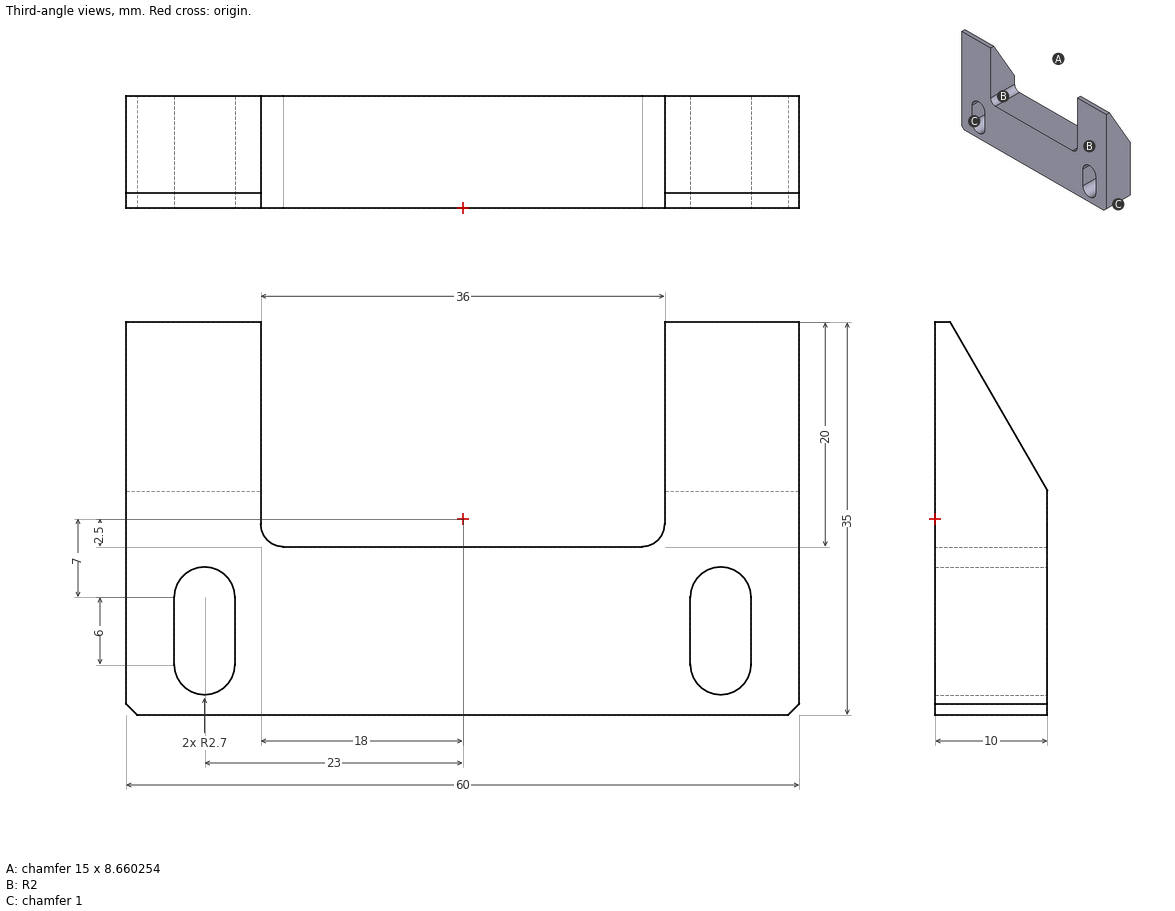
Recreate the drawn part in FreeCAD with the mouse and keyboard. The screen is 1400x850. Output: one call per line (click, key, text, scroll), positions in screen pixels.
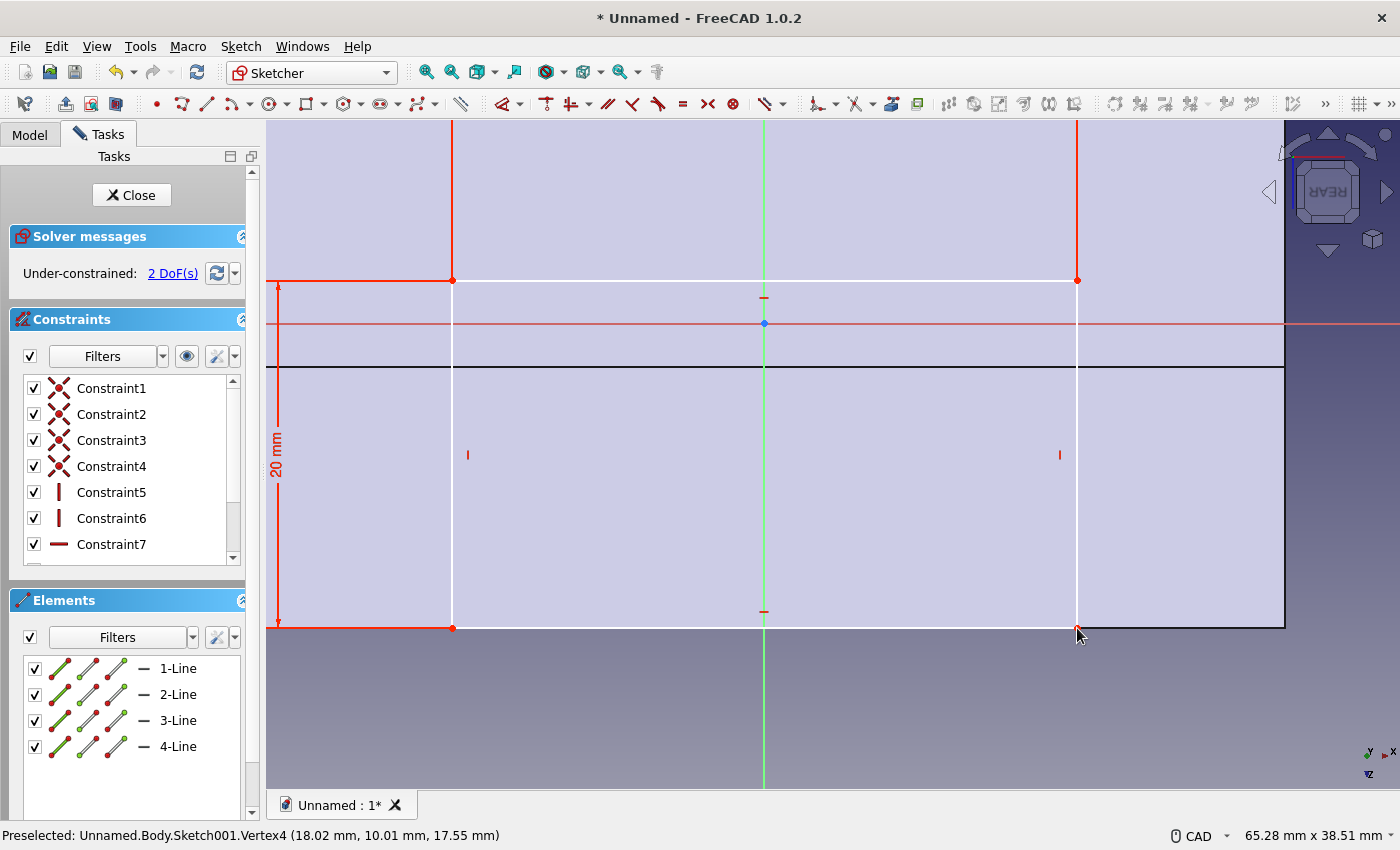
click(502, 104)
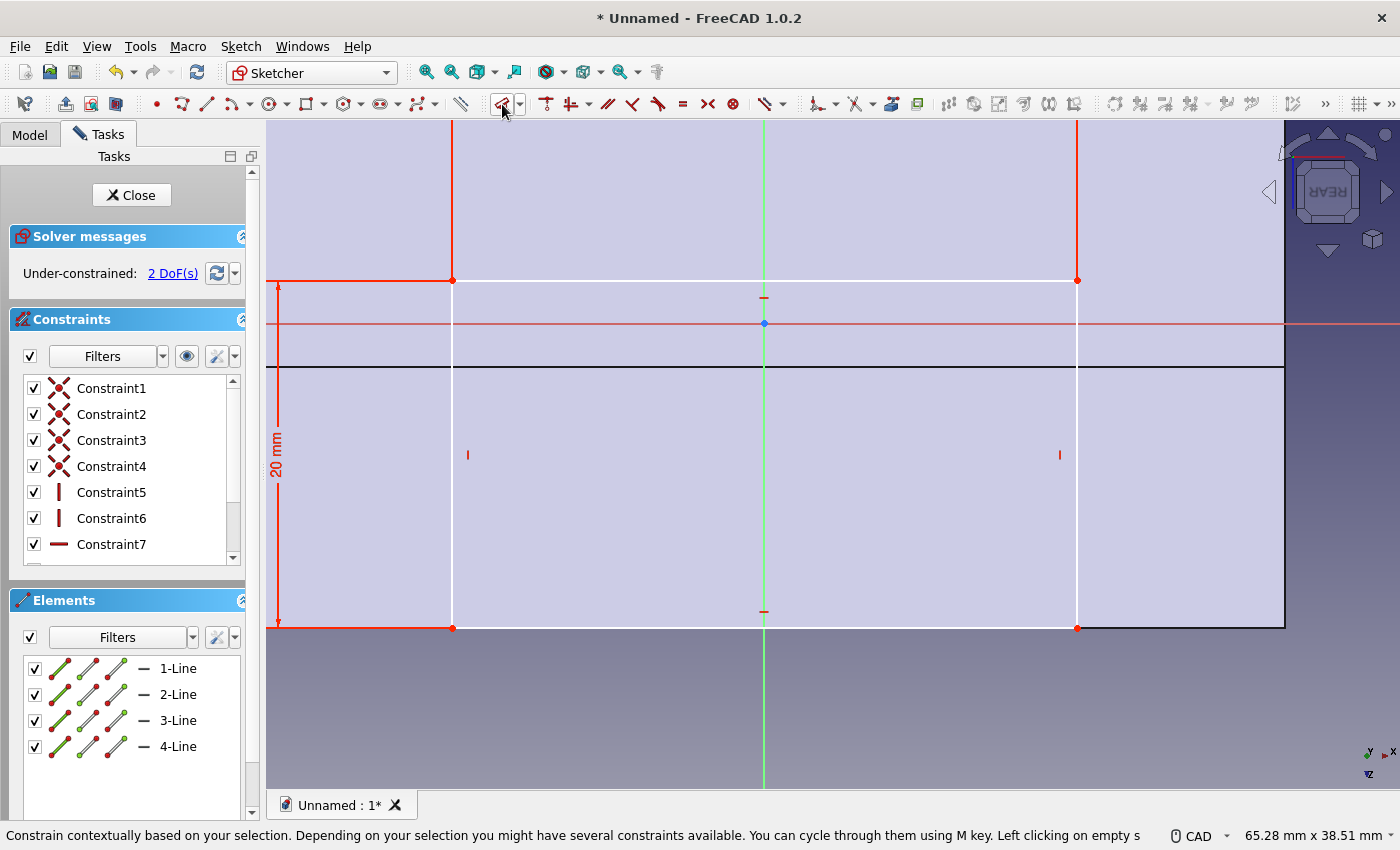
click(452, 281)
click(608, 247)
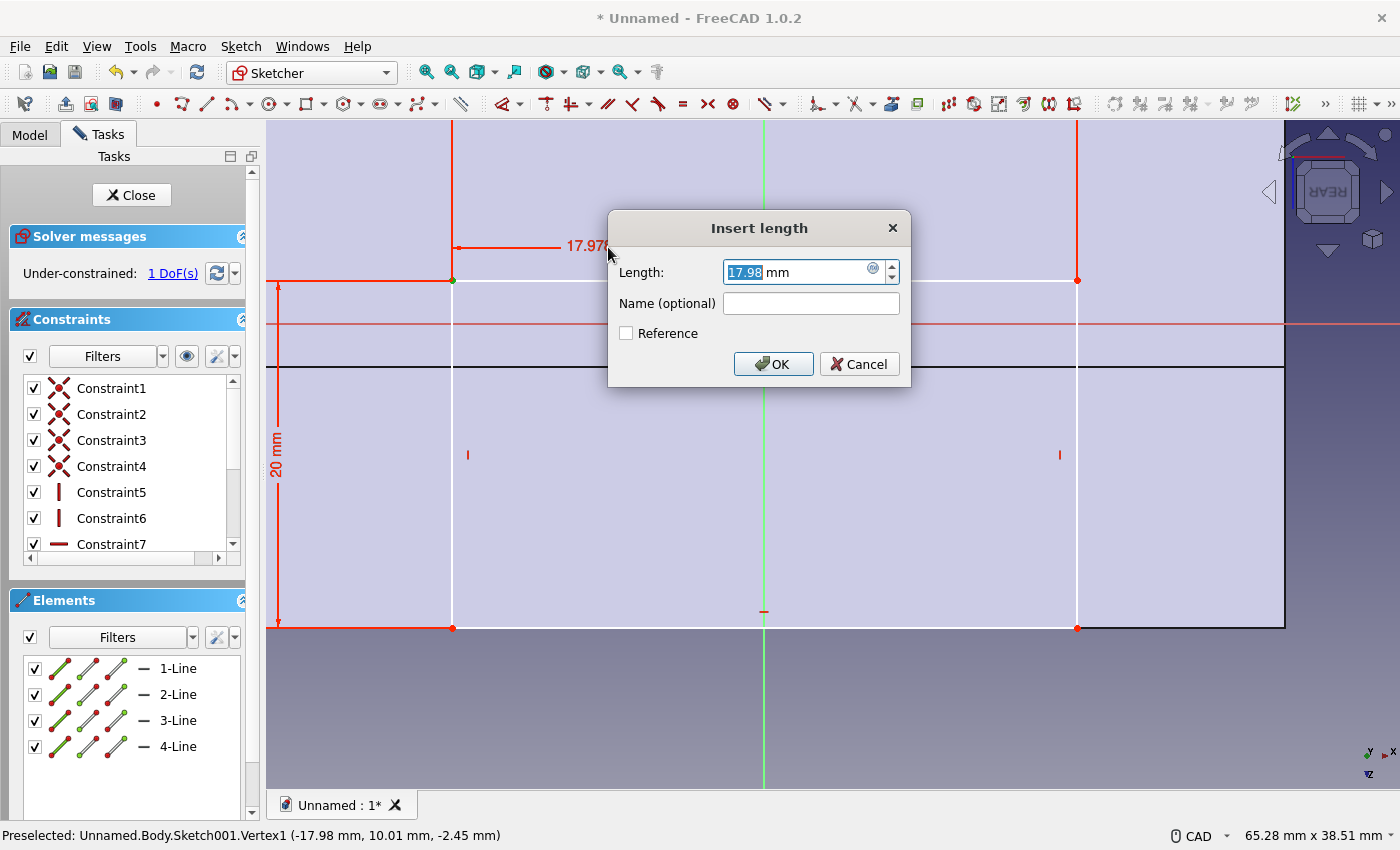
text(18)
key(Return)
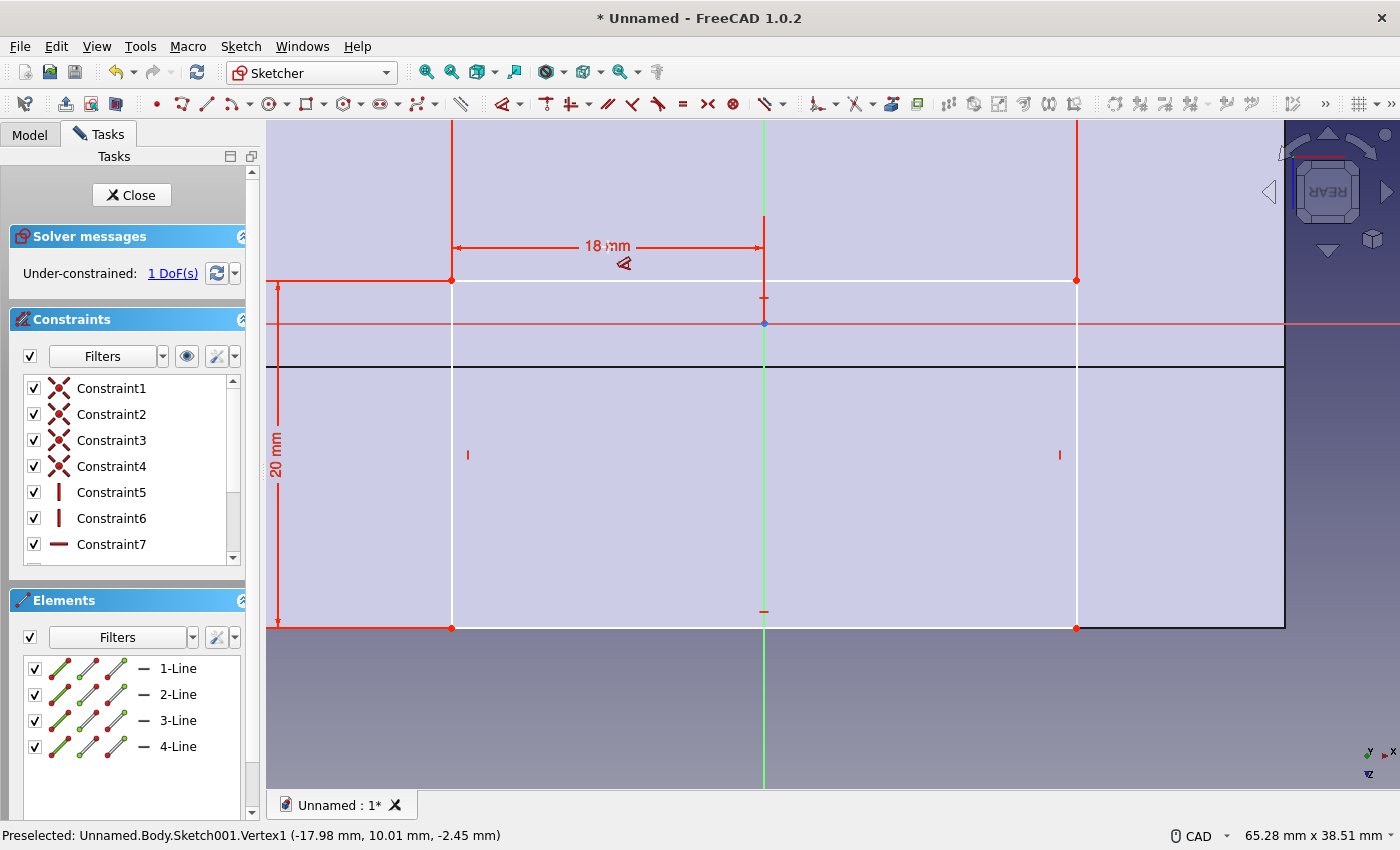
click(452, 281)
click(418, 302)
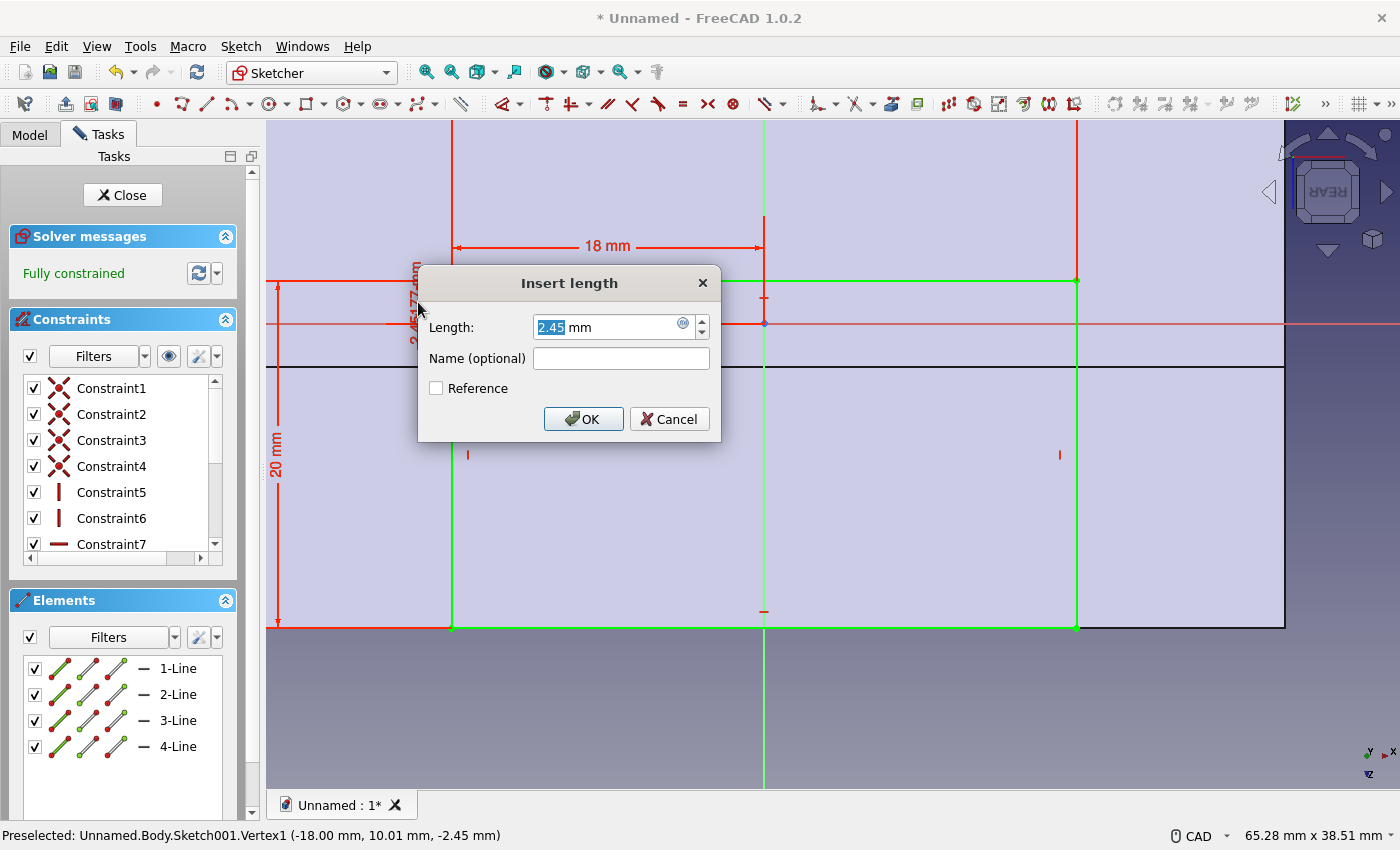
text(2.5)
key(Return)
key(Escape)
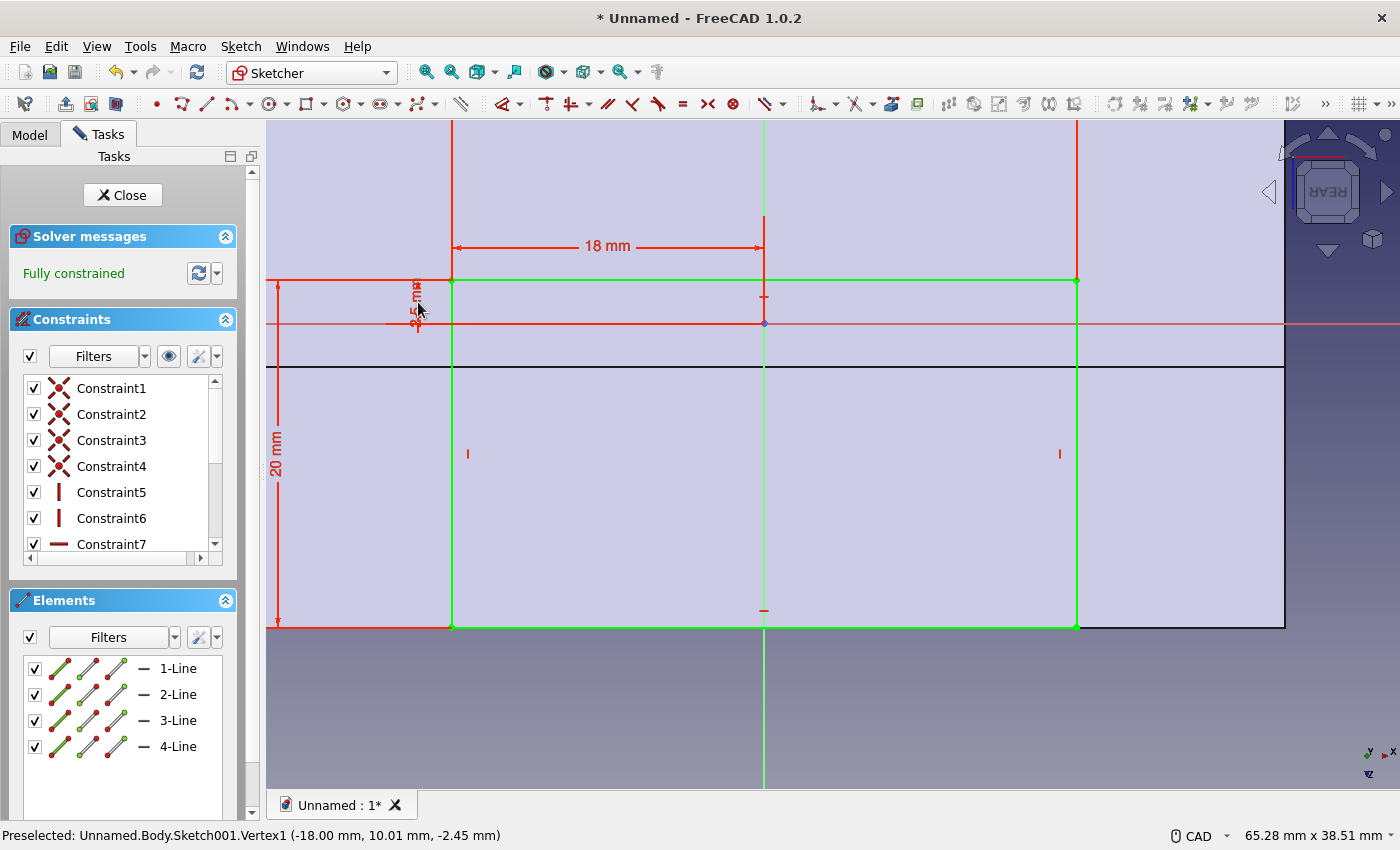
click(123, 195)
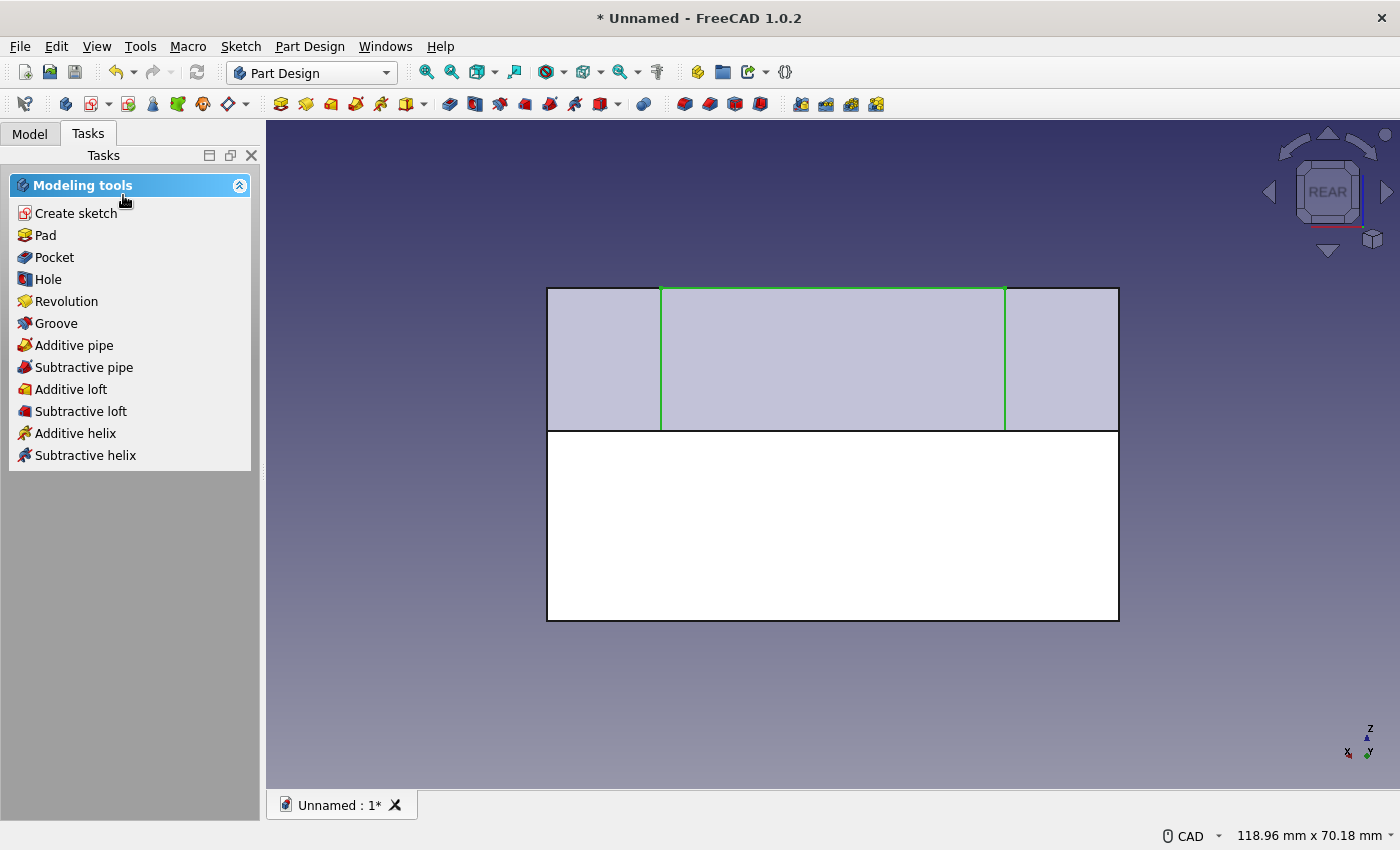
click(450, 104)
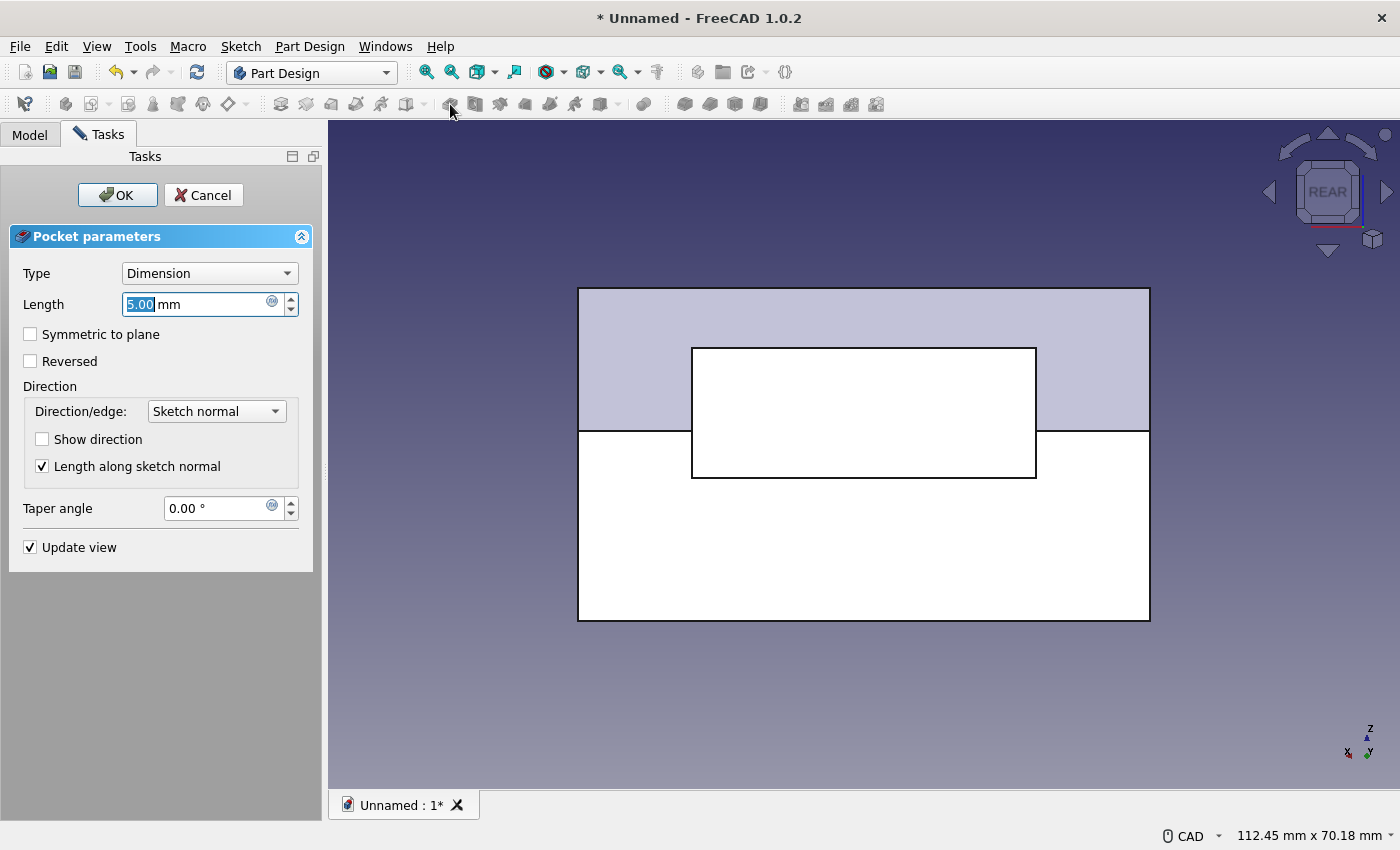
click(210, 274)